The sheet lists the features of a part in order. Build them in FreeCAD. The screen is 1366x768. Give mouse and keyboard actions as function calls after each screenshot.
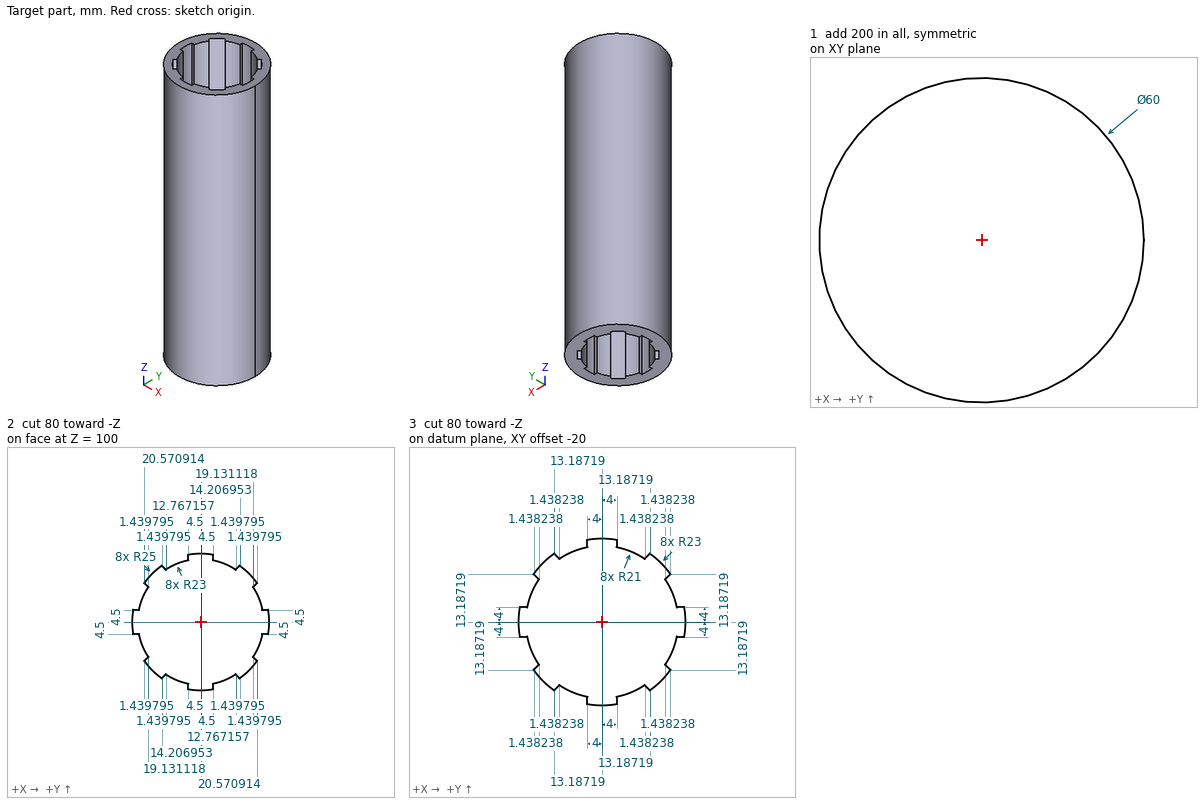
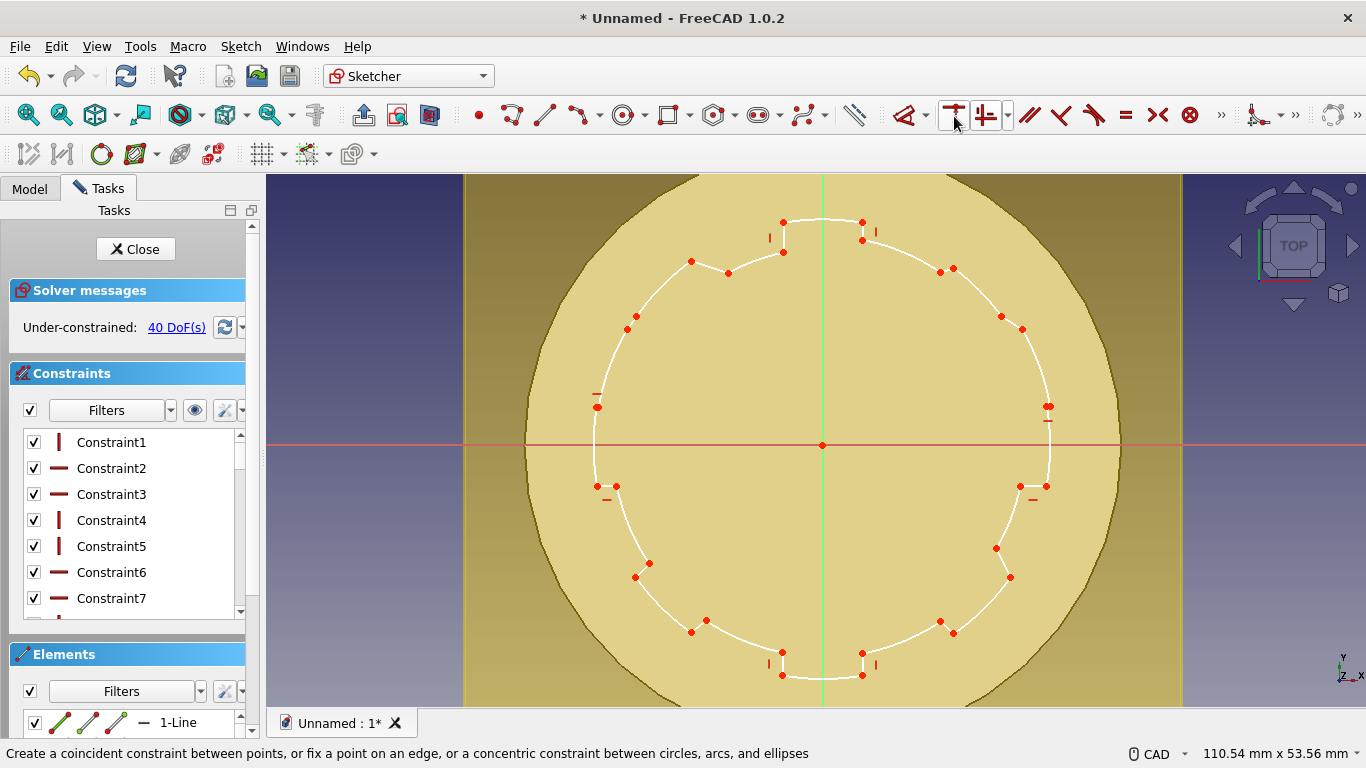
click(919, 260)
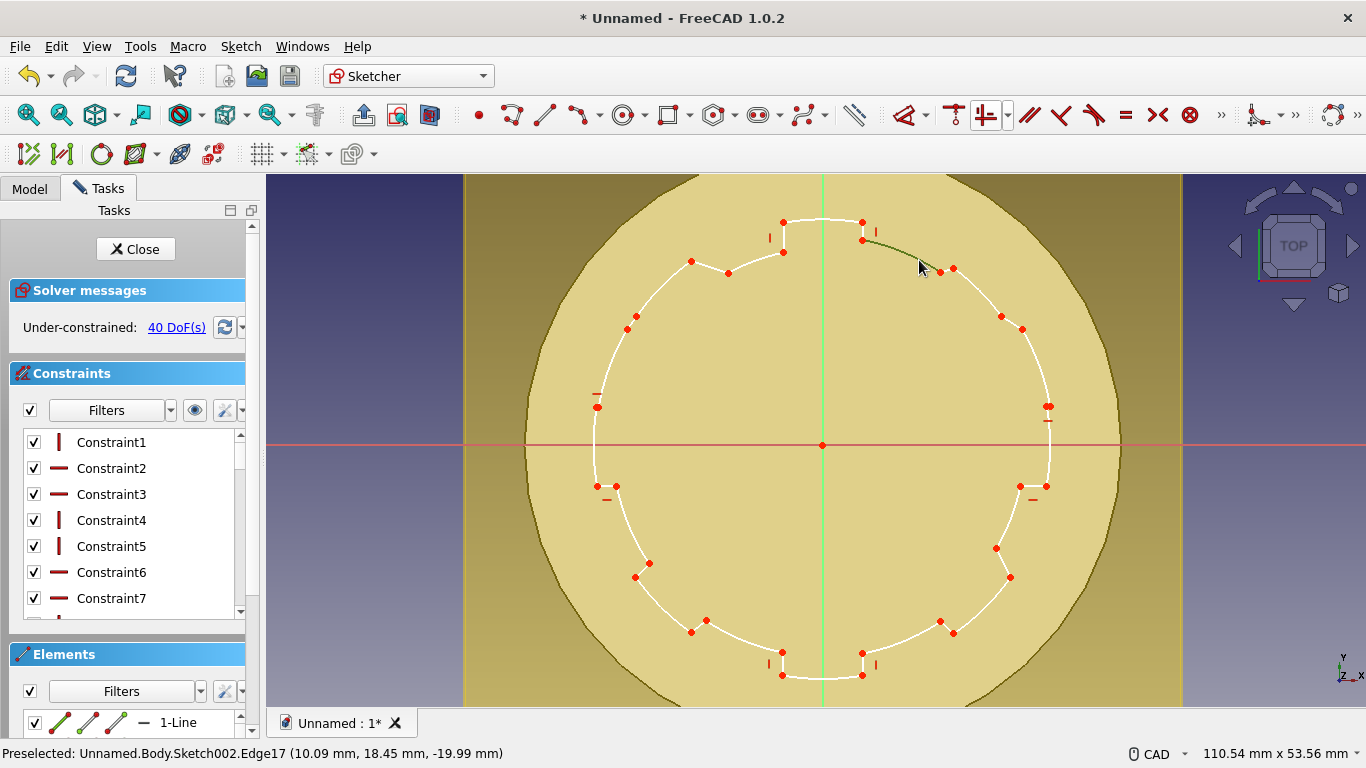
click(1045, 383)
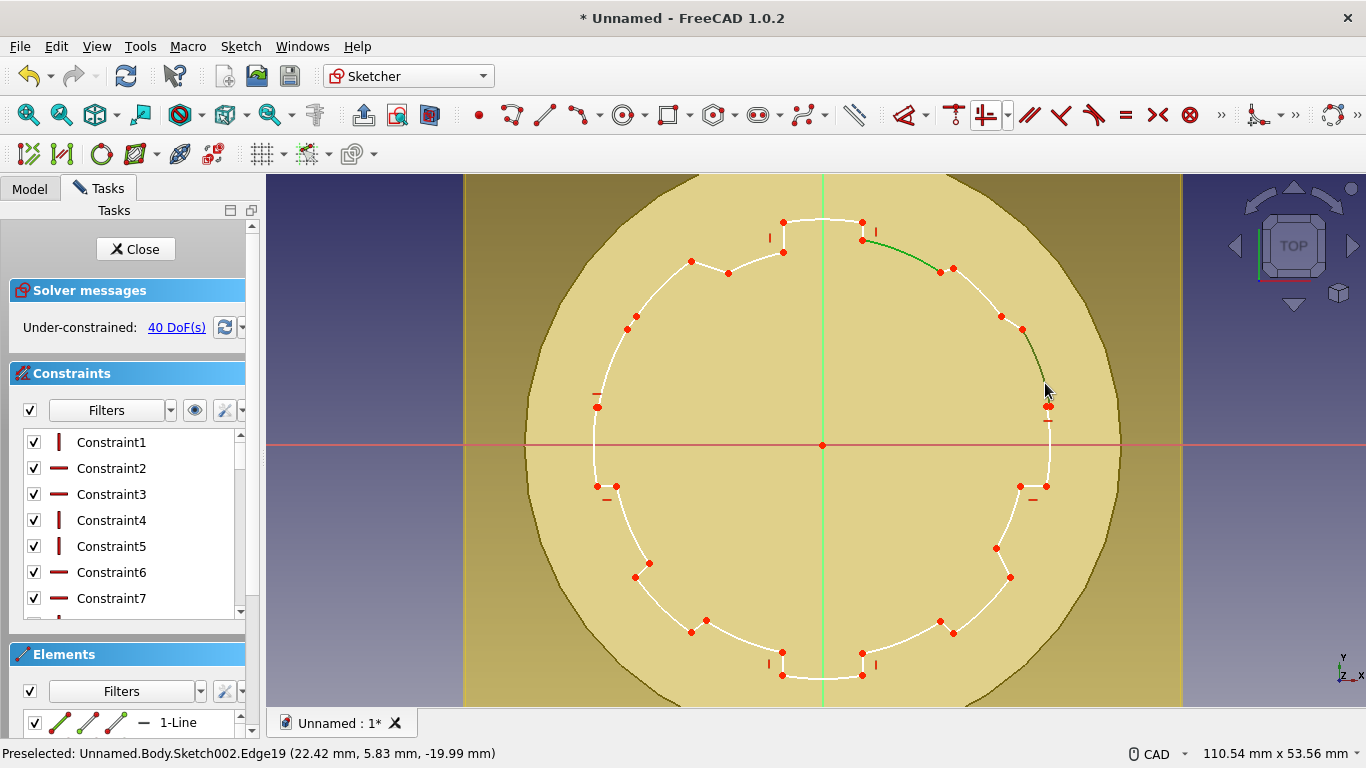
click(1006, 531)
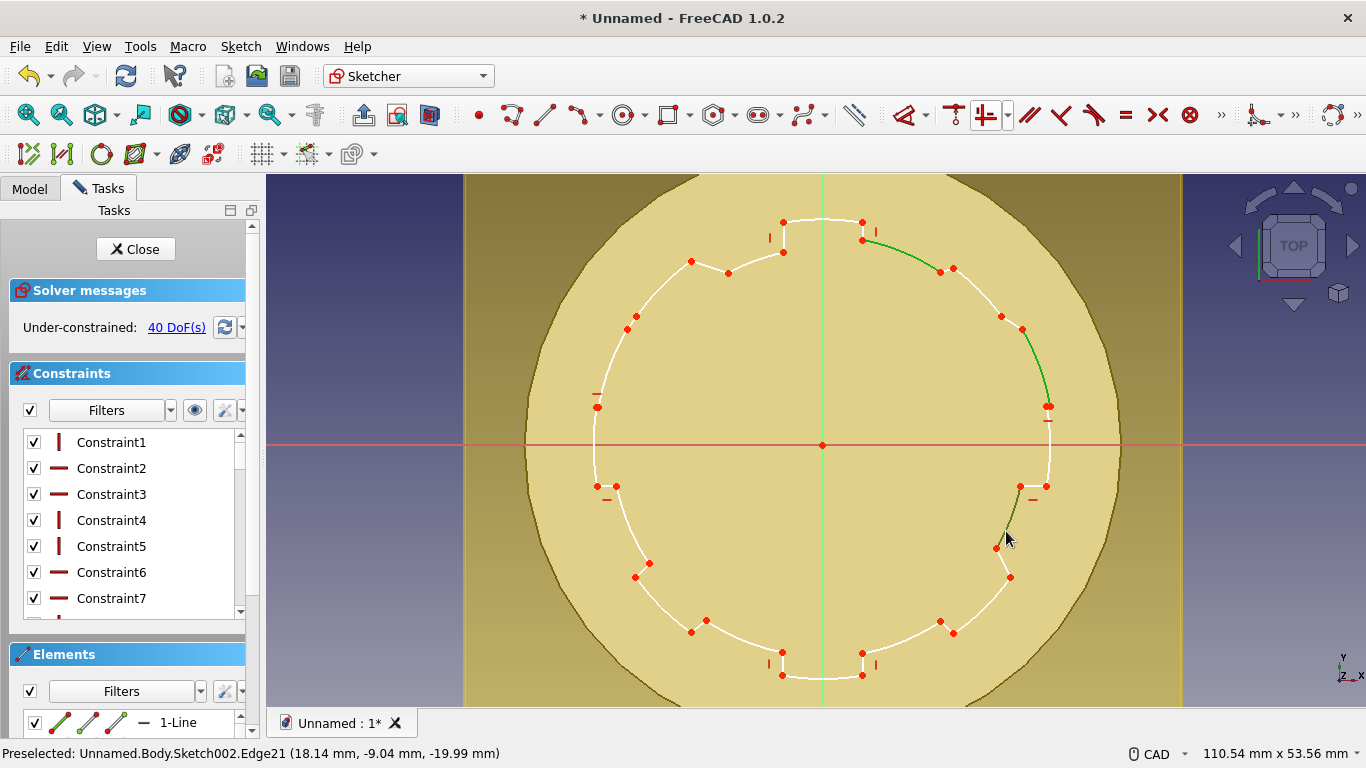
click(887, 647)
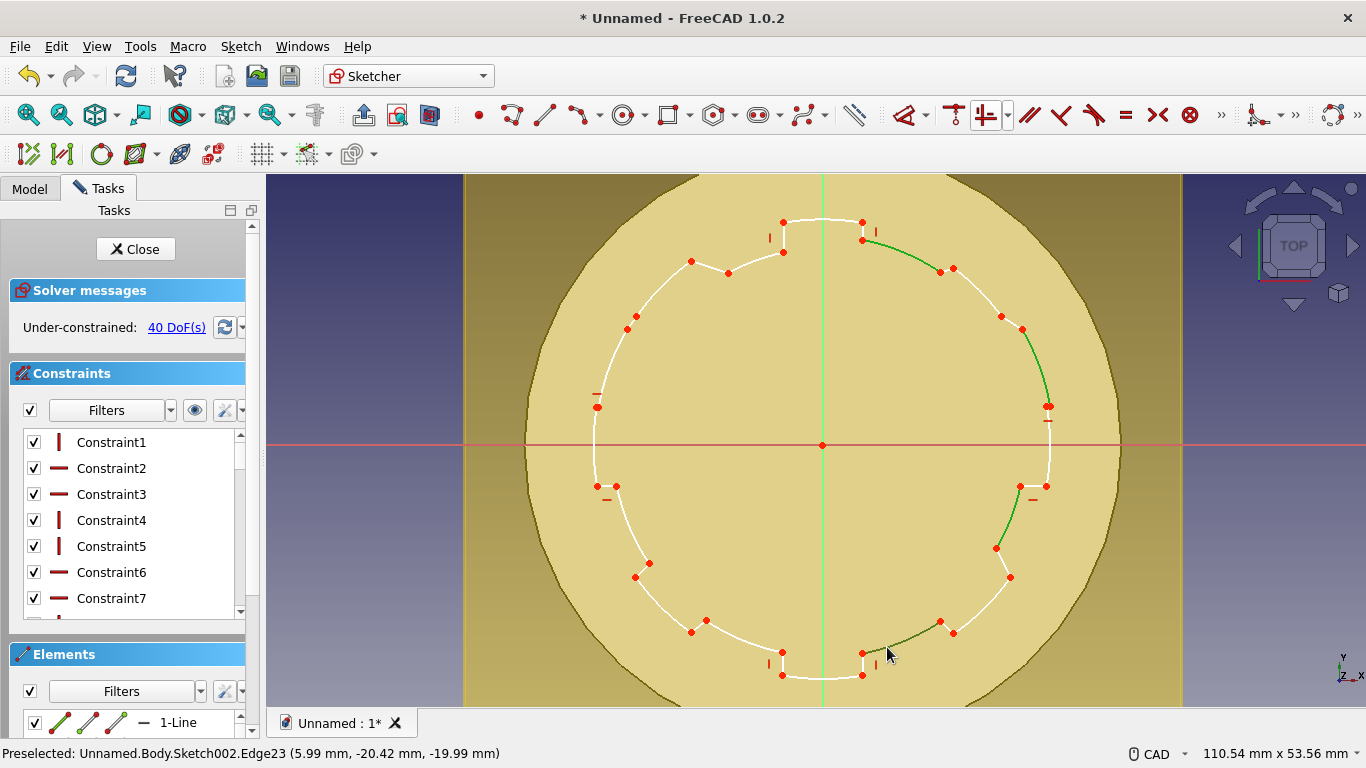
click(728, 633)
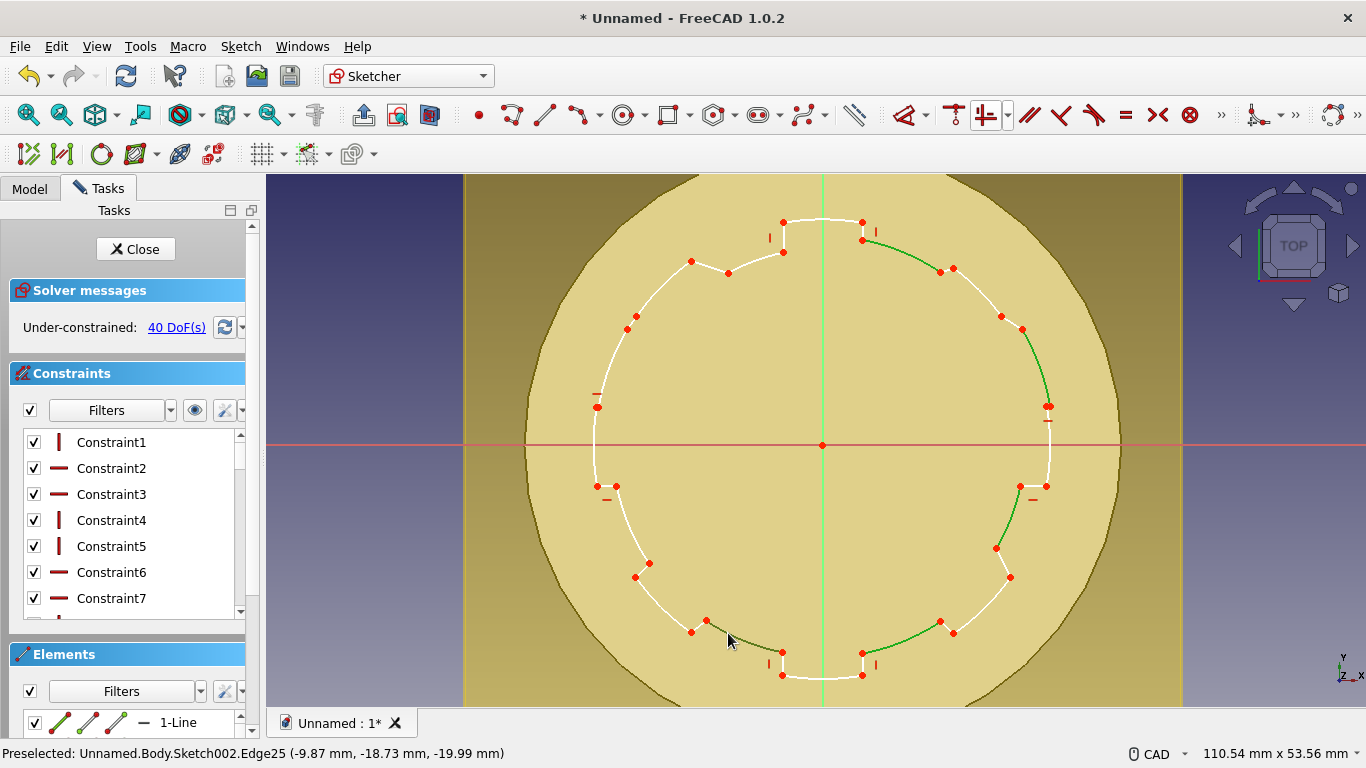
click(623, 511)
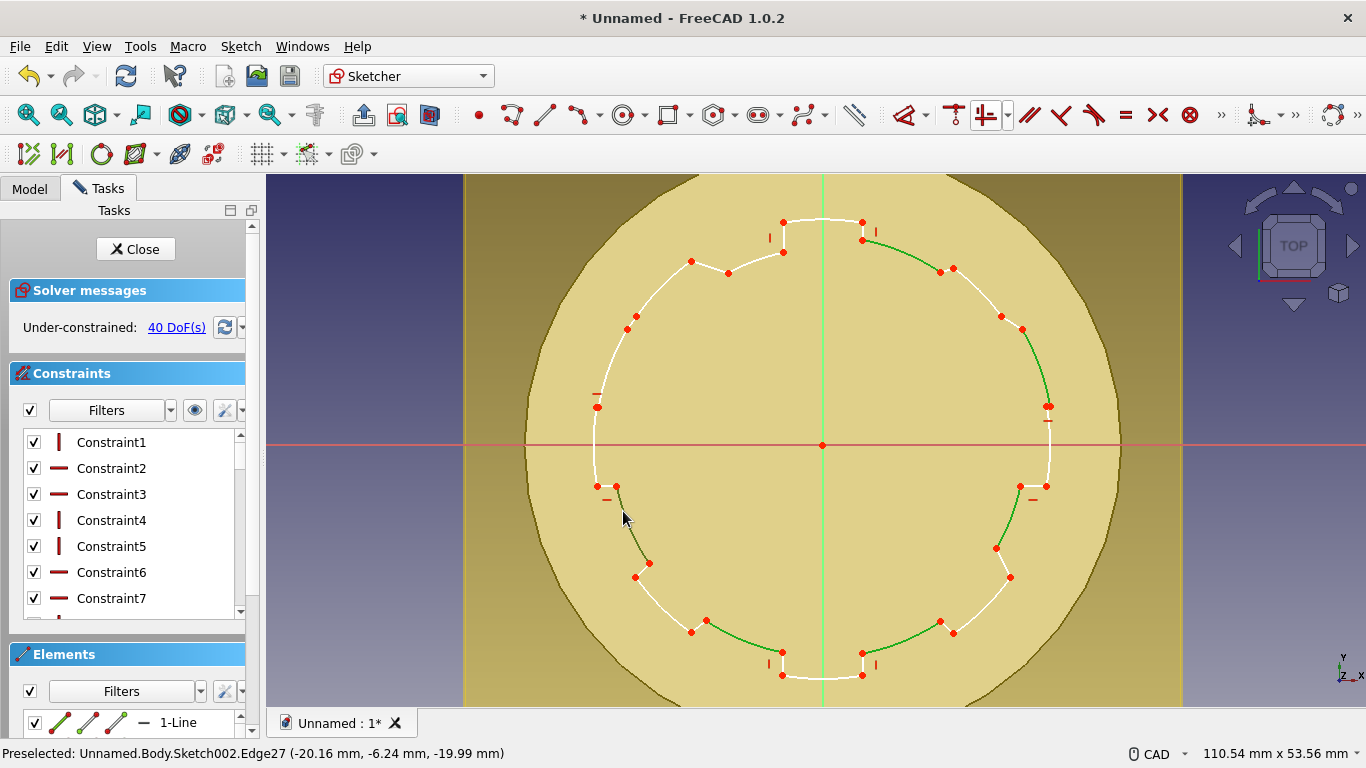
click(616, 352)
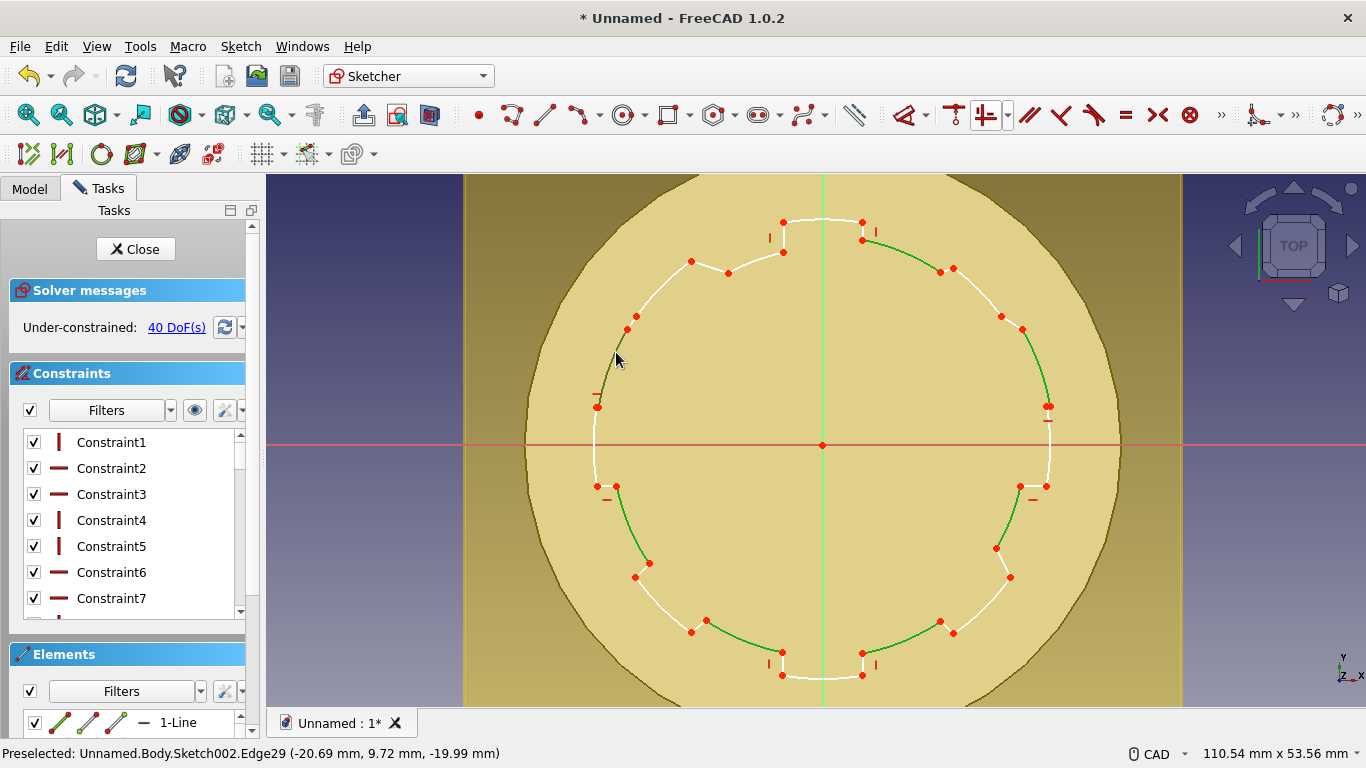
click(767, 257)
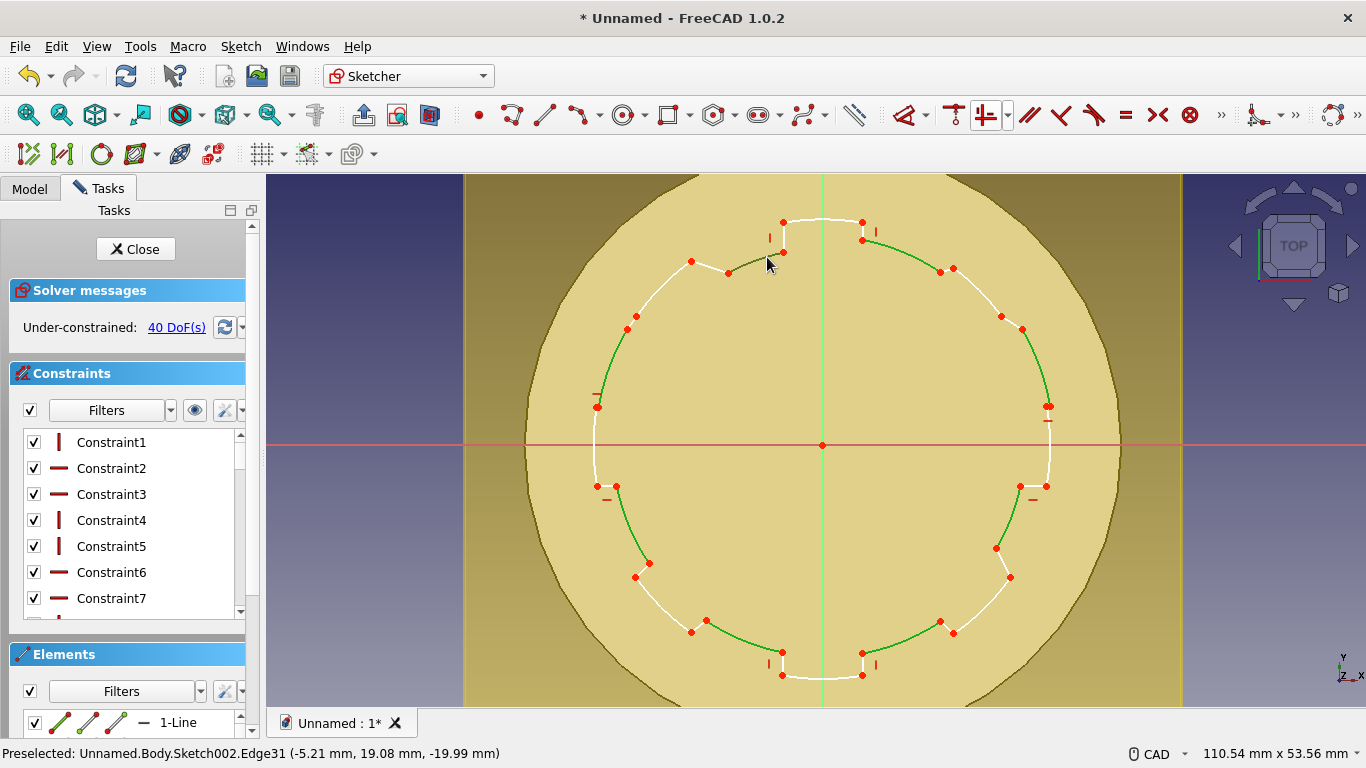
click(1126, 116)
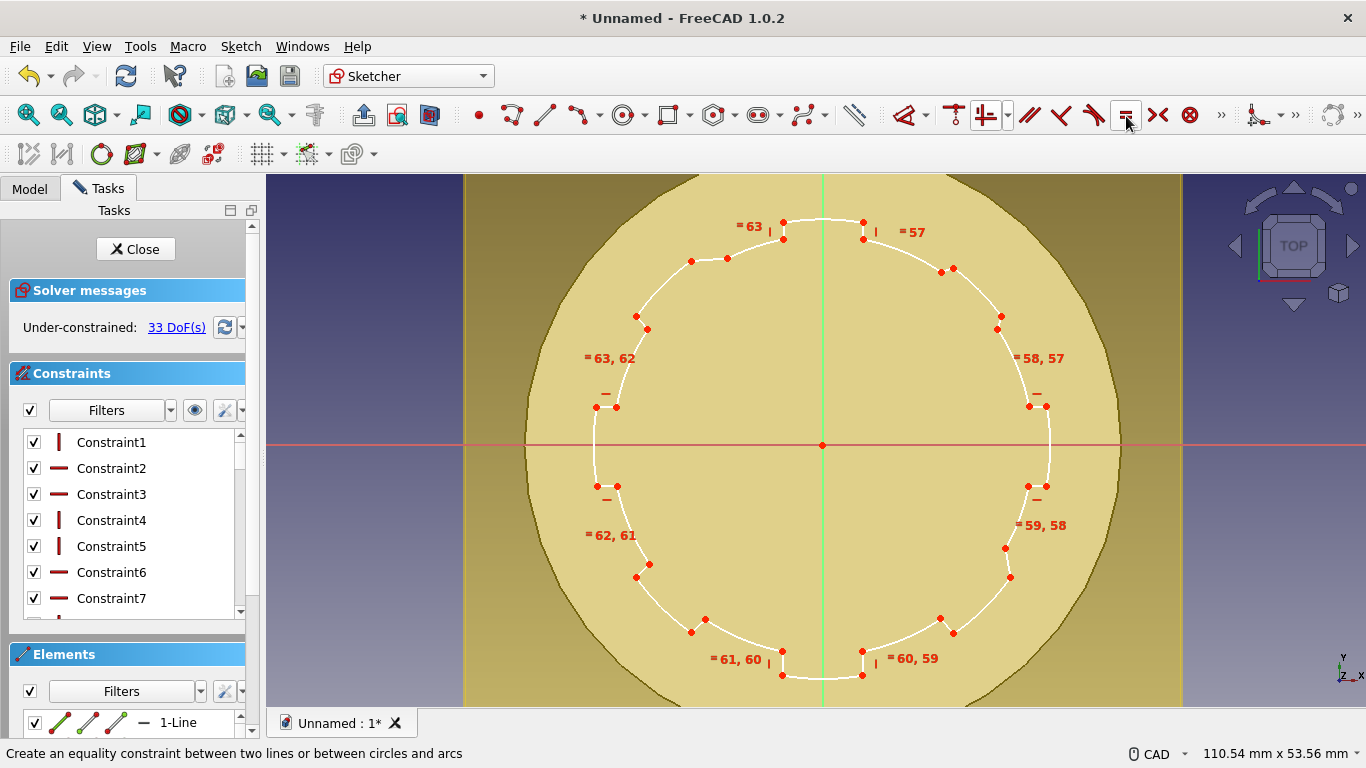
click(989, 300)